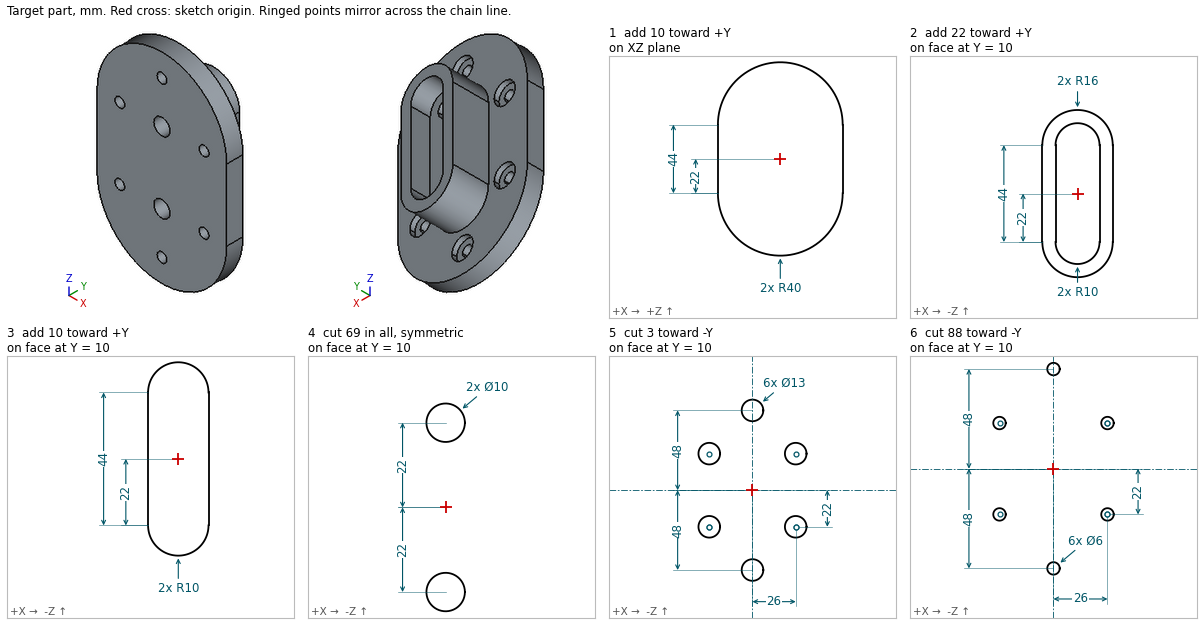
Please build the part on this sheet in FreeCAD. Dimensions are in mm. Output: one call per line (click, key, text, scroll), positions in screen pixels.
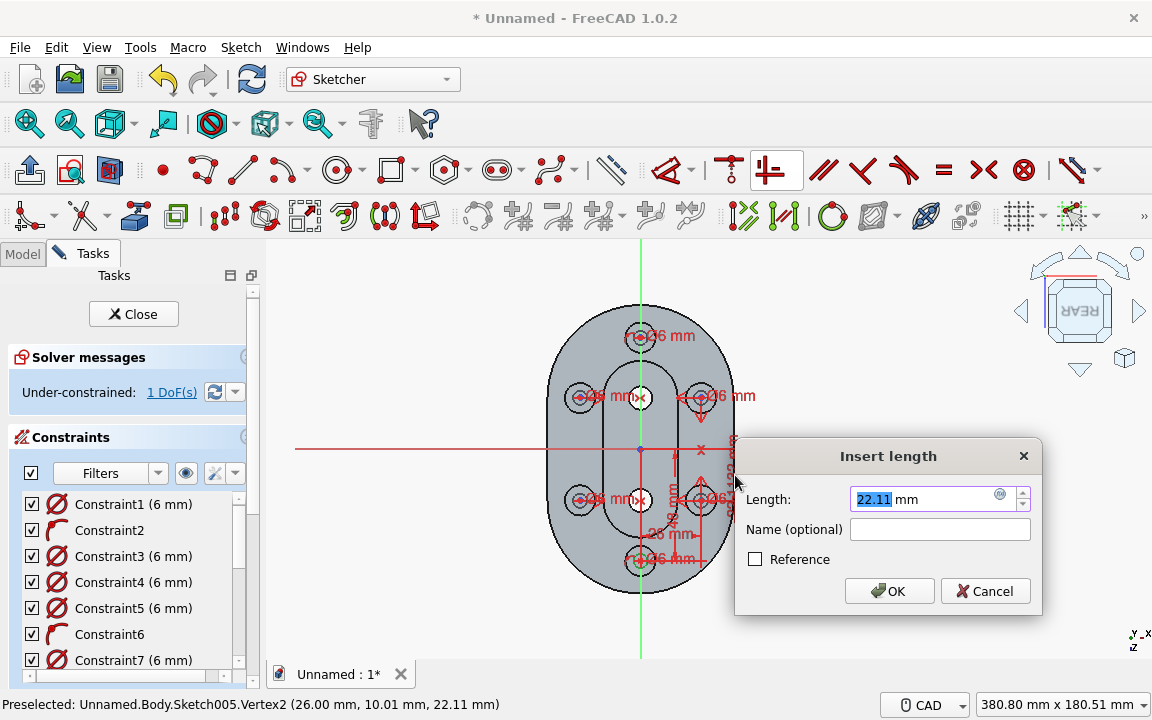
text(22)
key(Return)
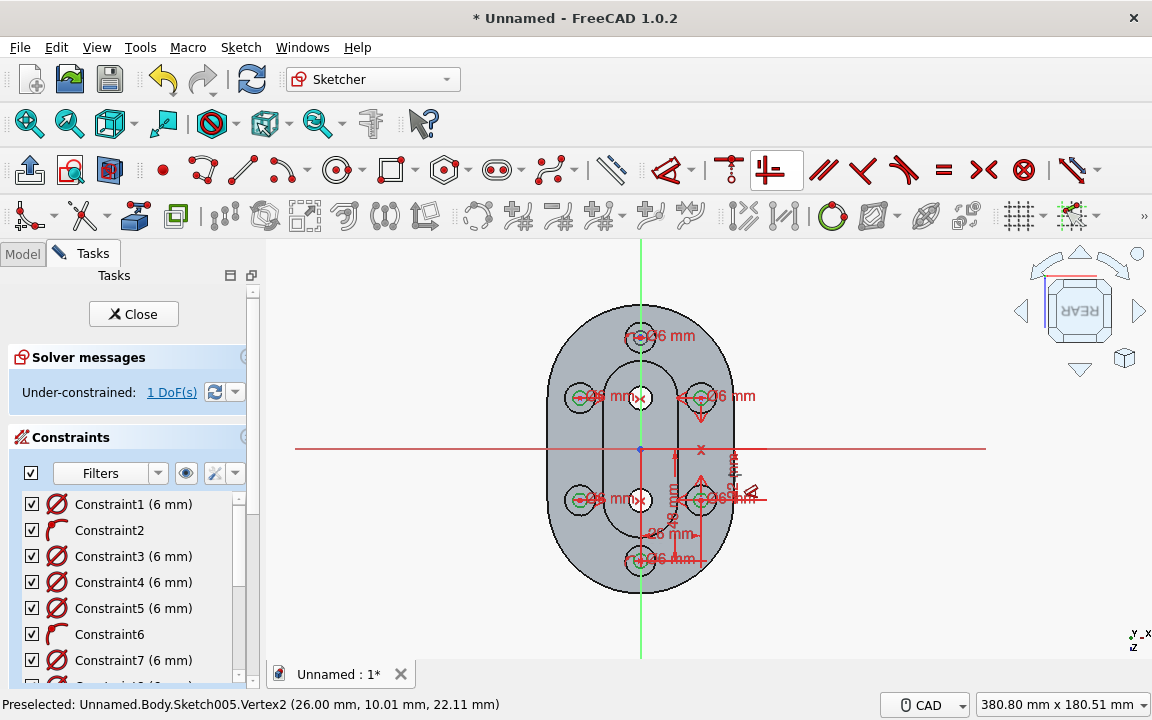
click(641, 338)
click(675, 394)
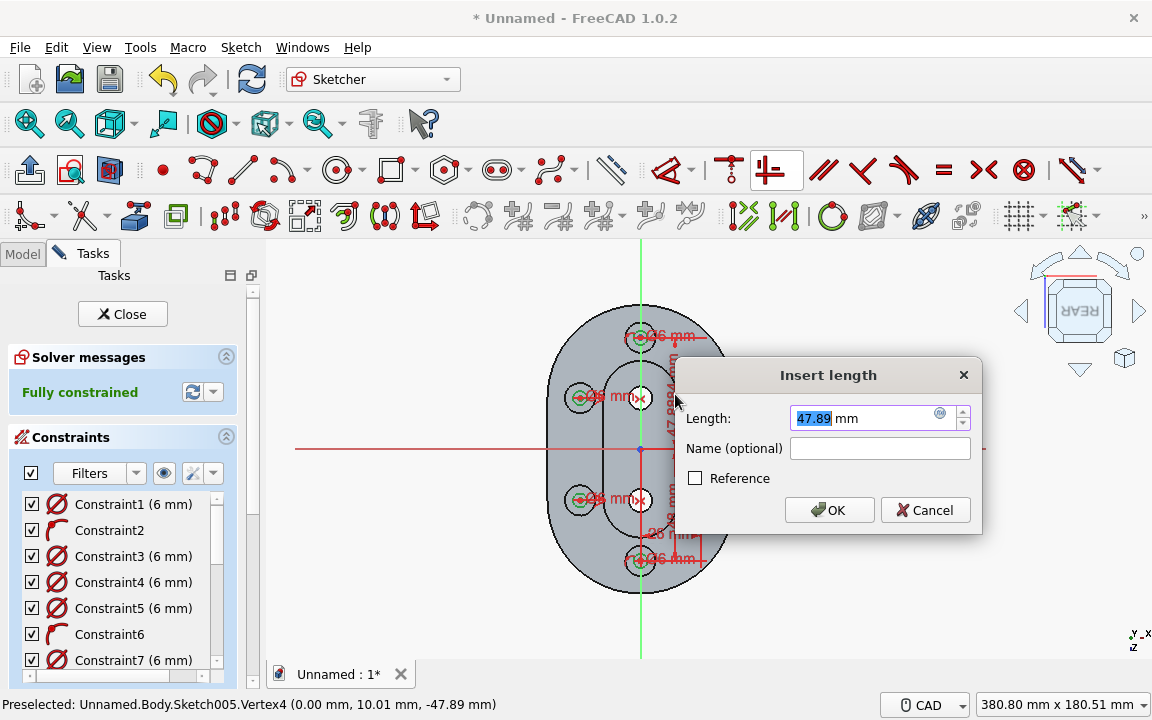
text(48)
key(Return)
key(Escape)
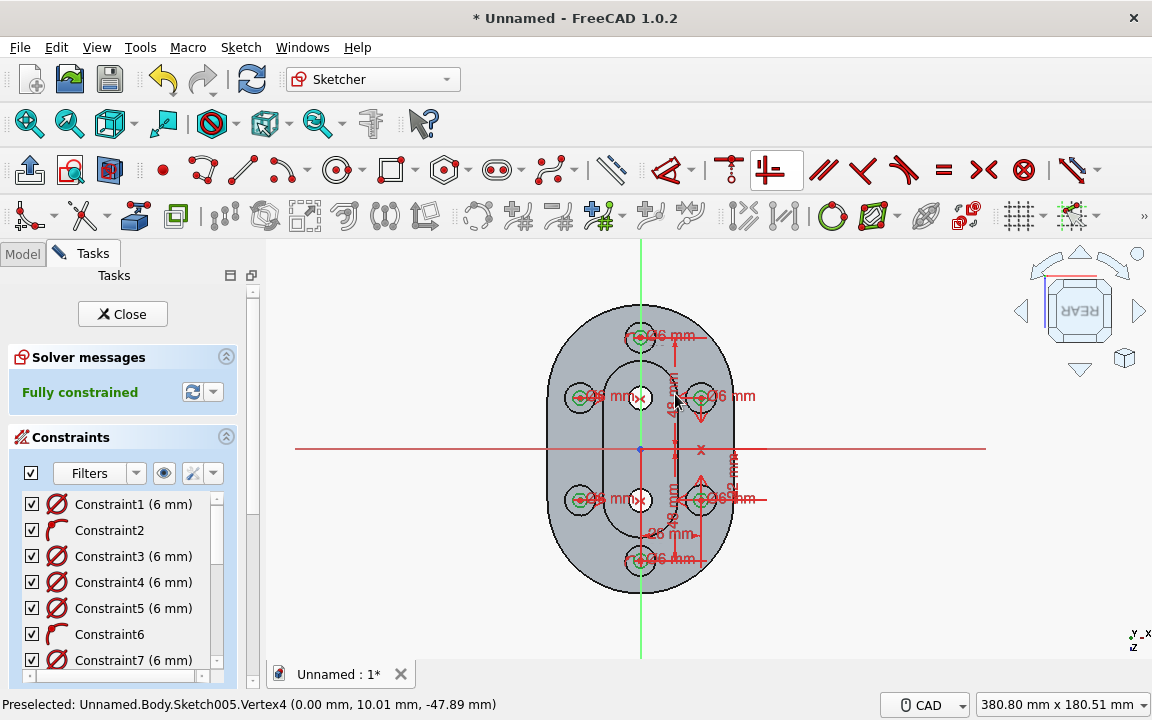
click(123, 314)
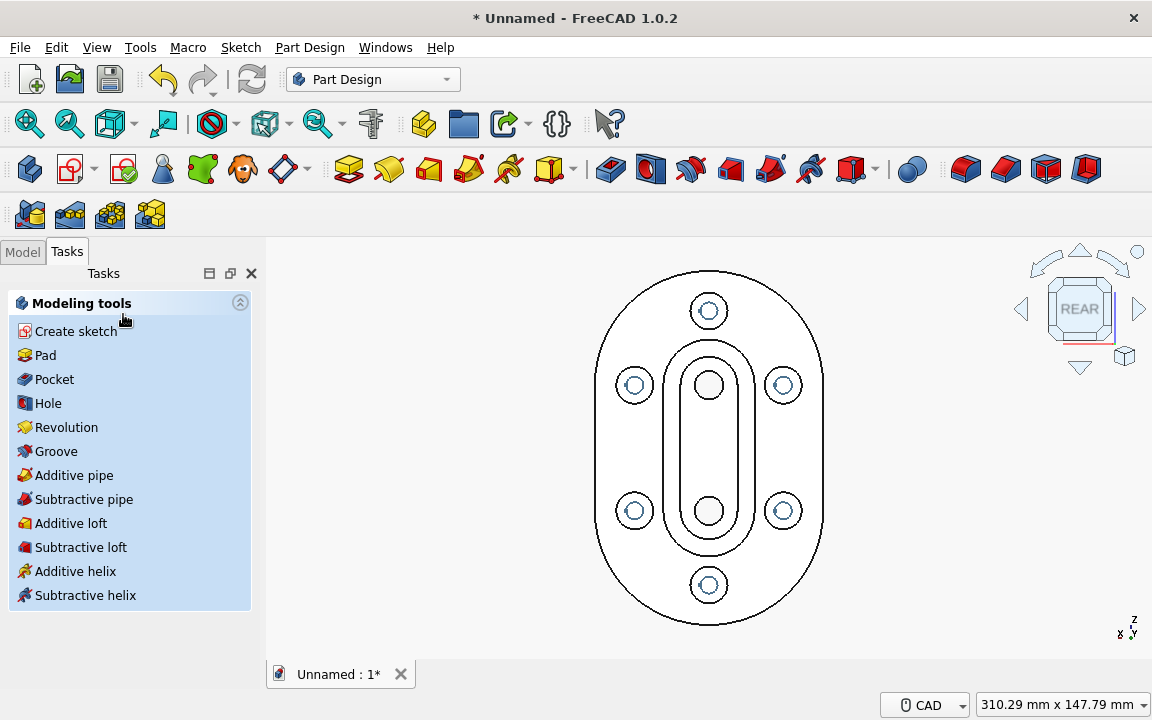
click(612, 170)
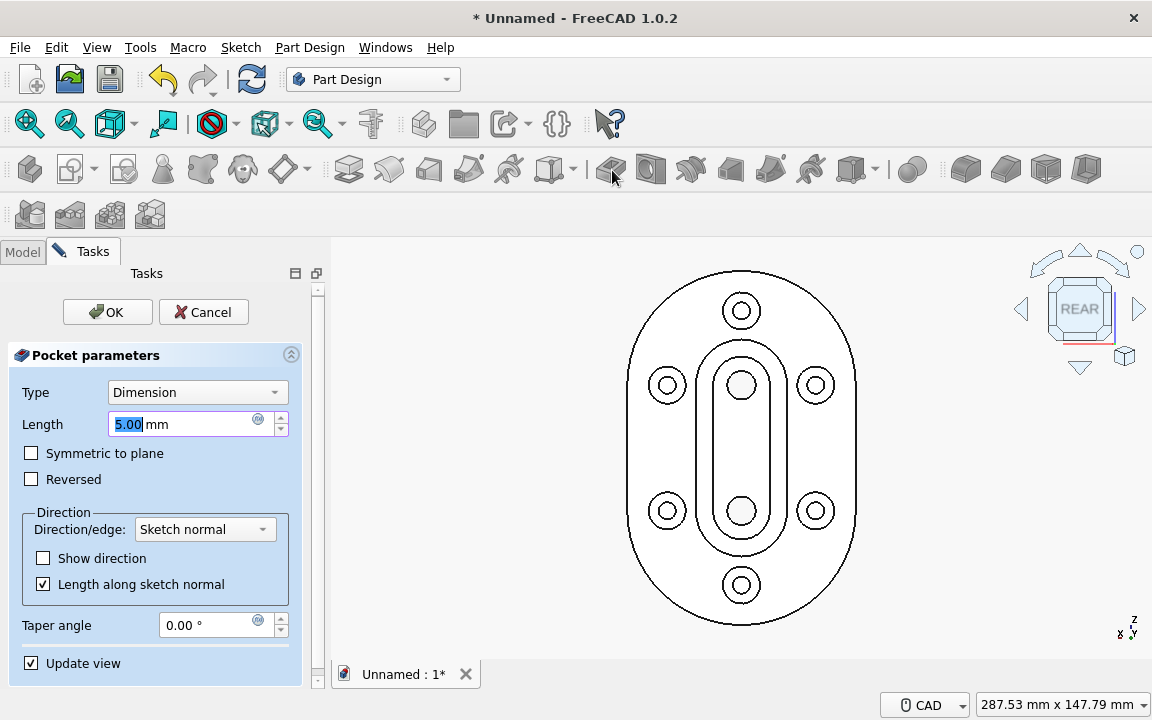
text(88)
key(Tab)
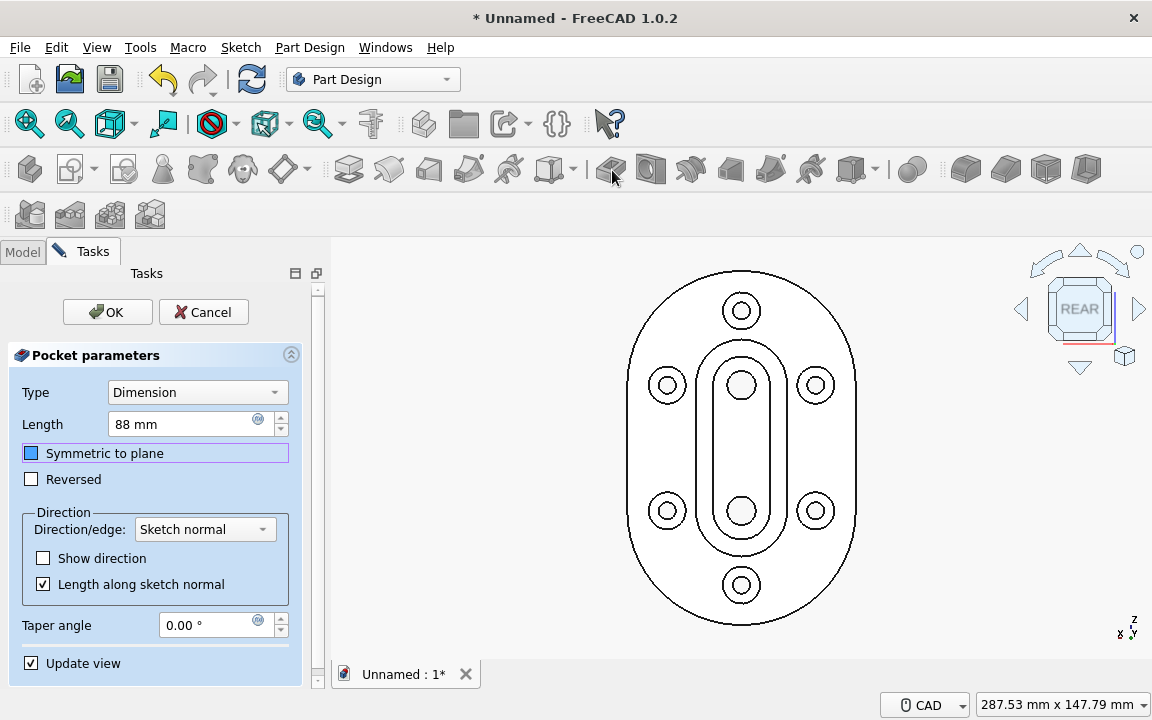
click(108, 312)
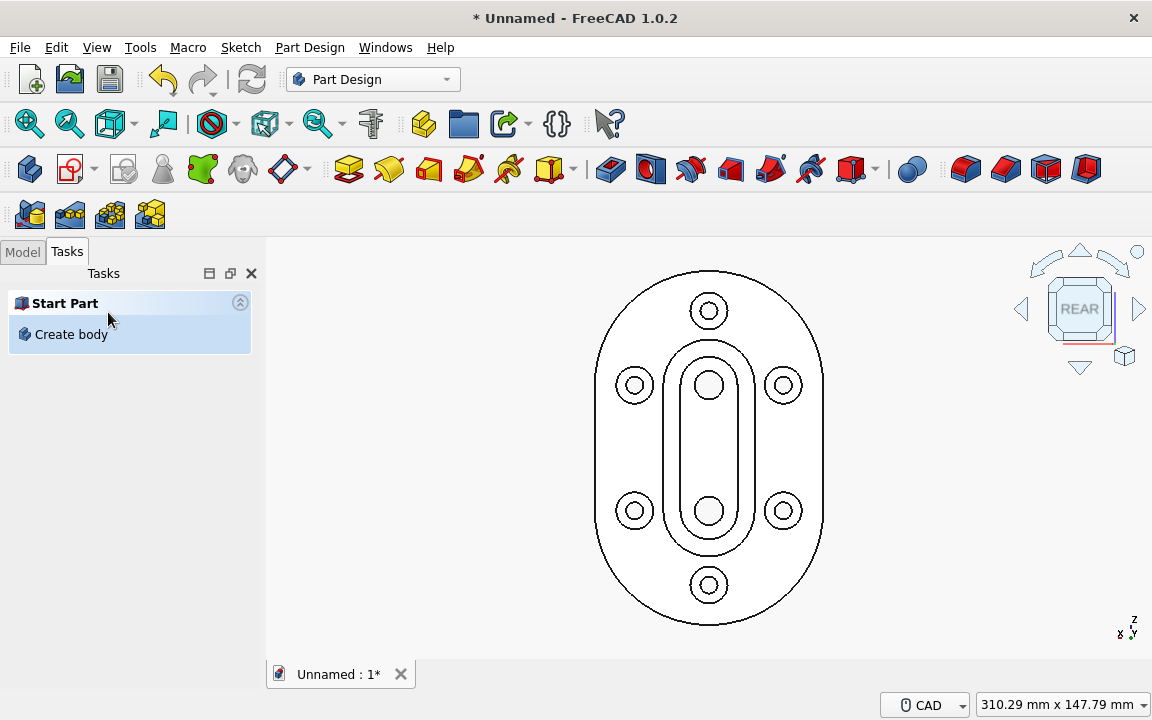
key(0)